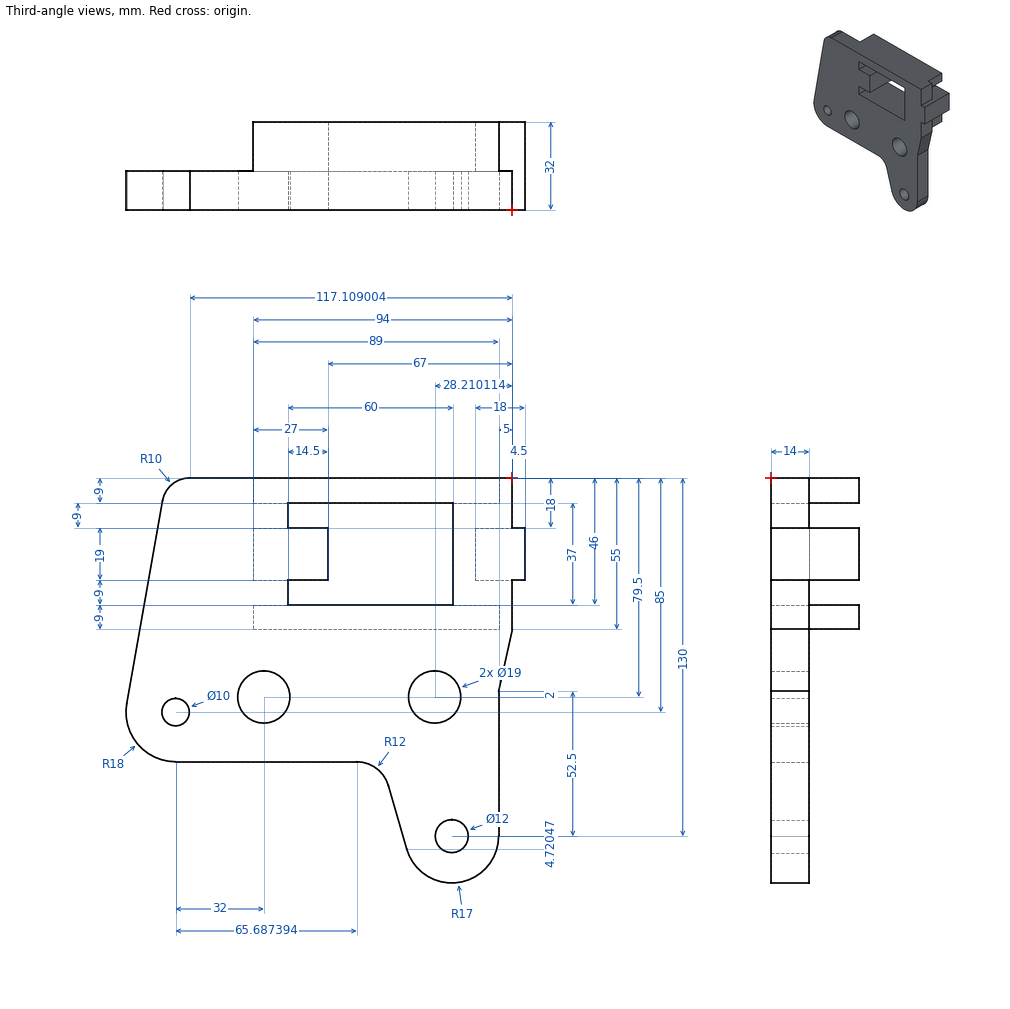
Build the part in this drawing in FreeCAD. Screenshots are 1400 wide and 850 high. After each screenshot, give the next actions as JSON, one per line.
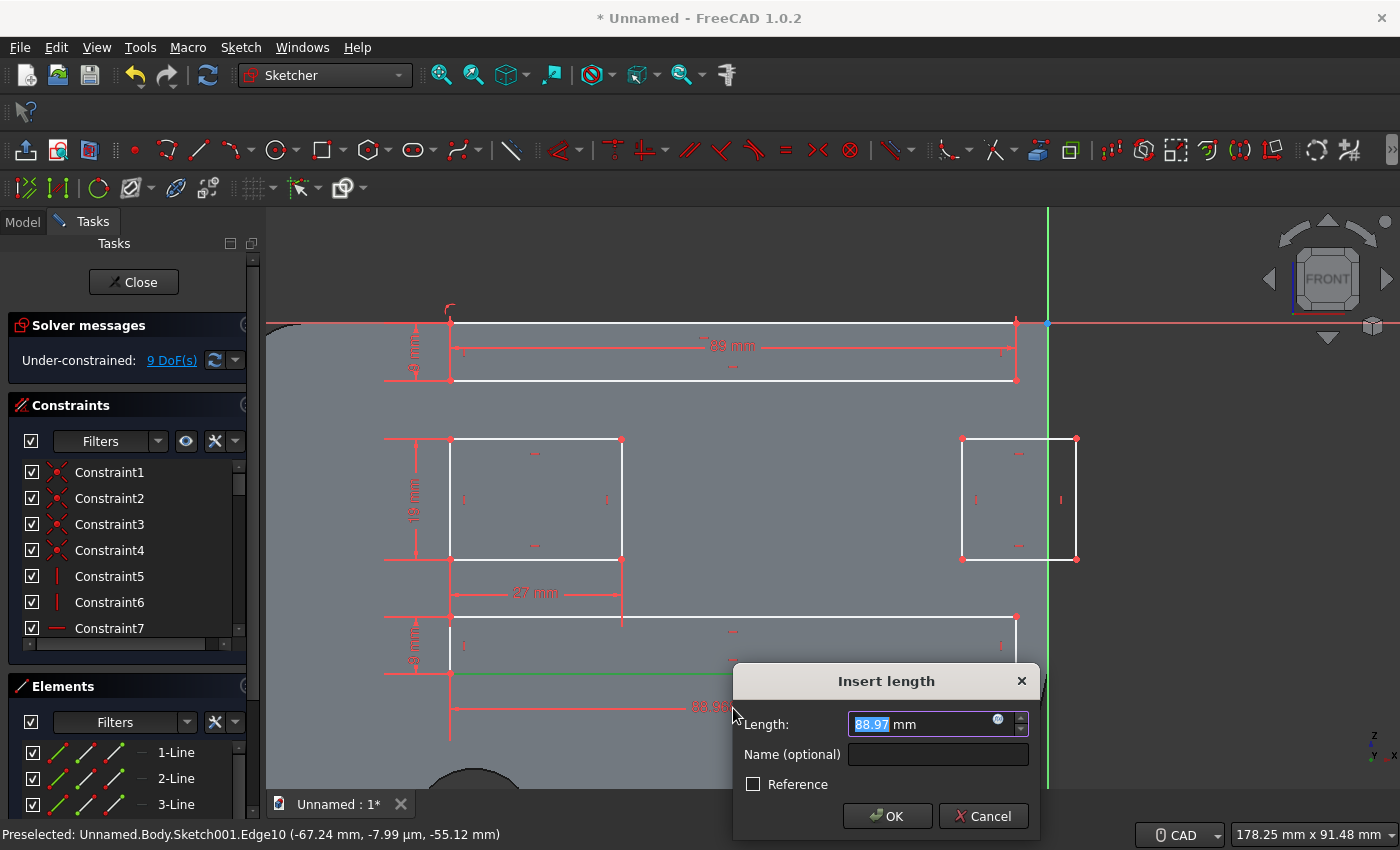
{"action": "type", "text": "89"}
{"action": "key", "text": "Return"}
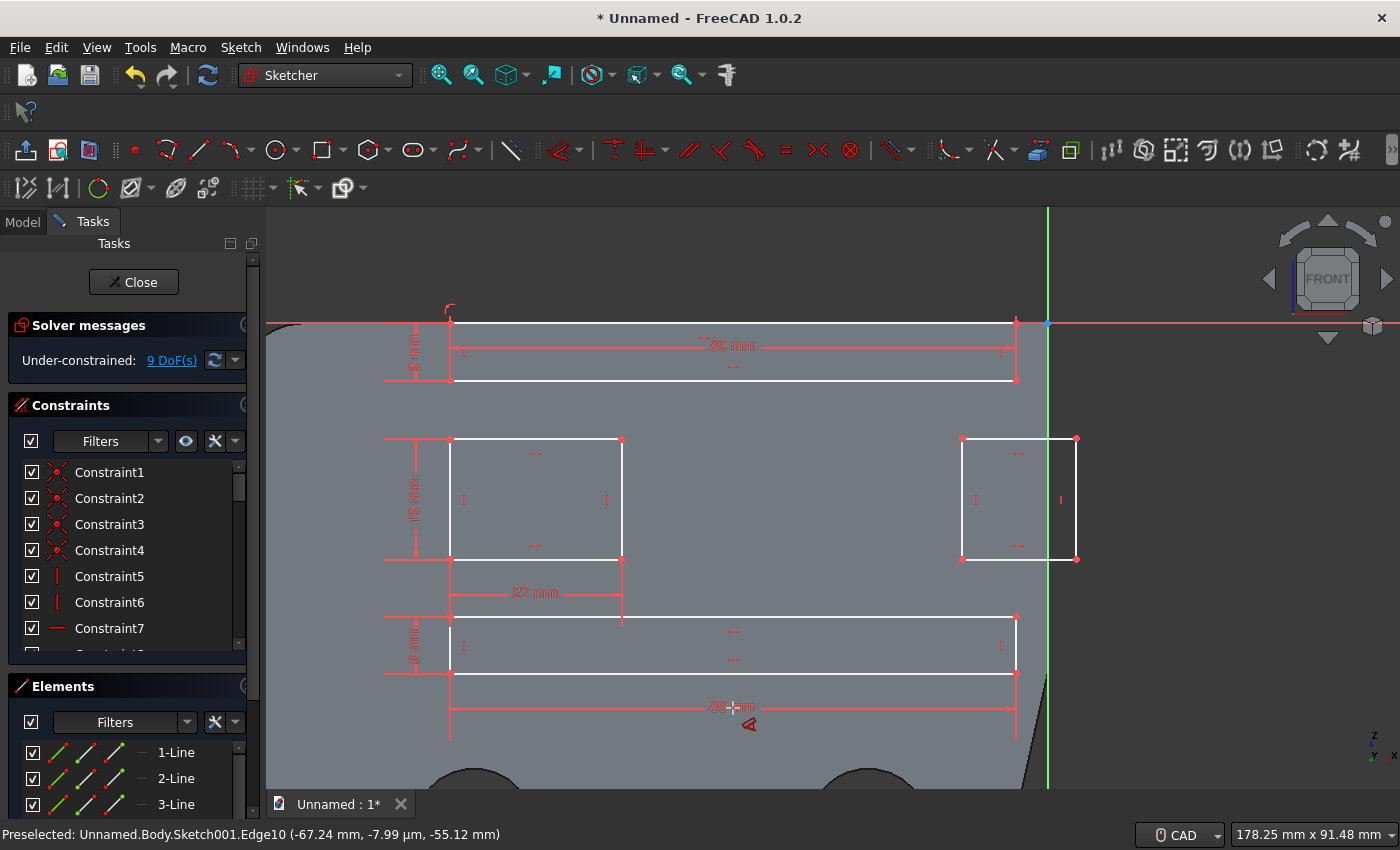
{"action": "left_click", "coordinate": [962, 475]}
{"action": "left_click", "coordinate": [996, 500]}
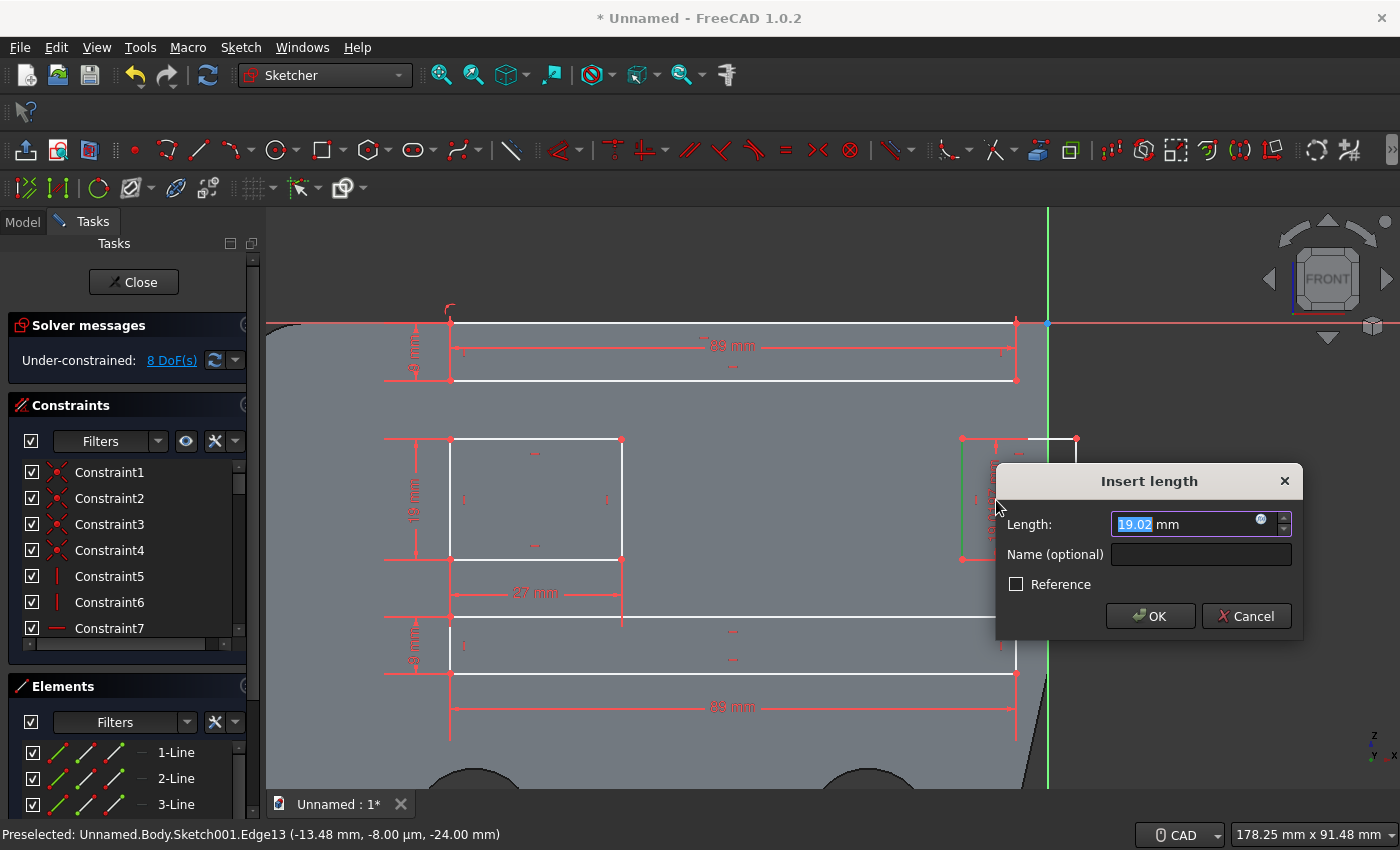
{"action": "type", "text": "19"}
{"action": "key", "text": "Return"}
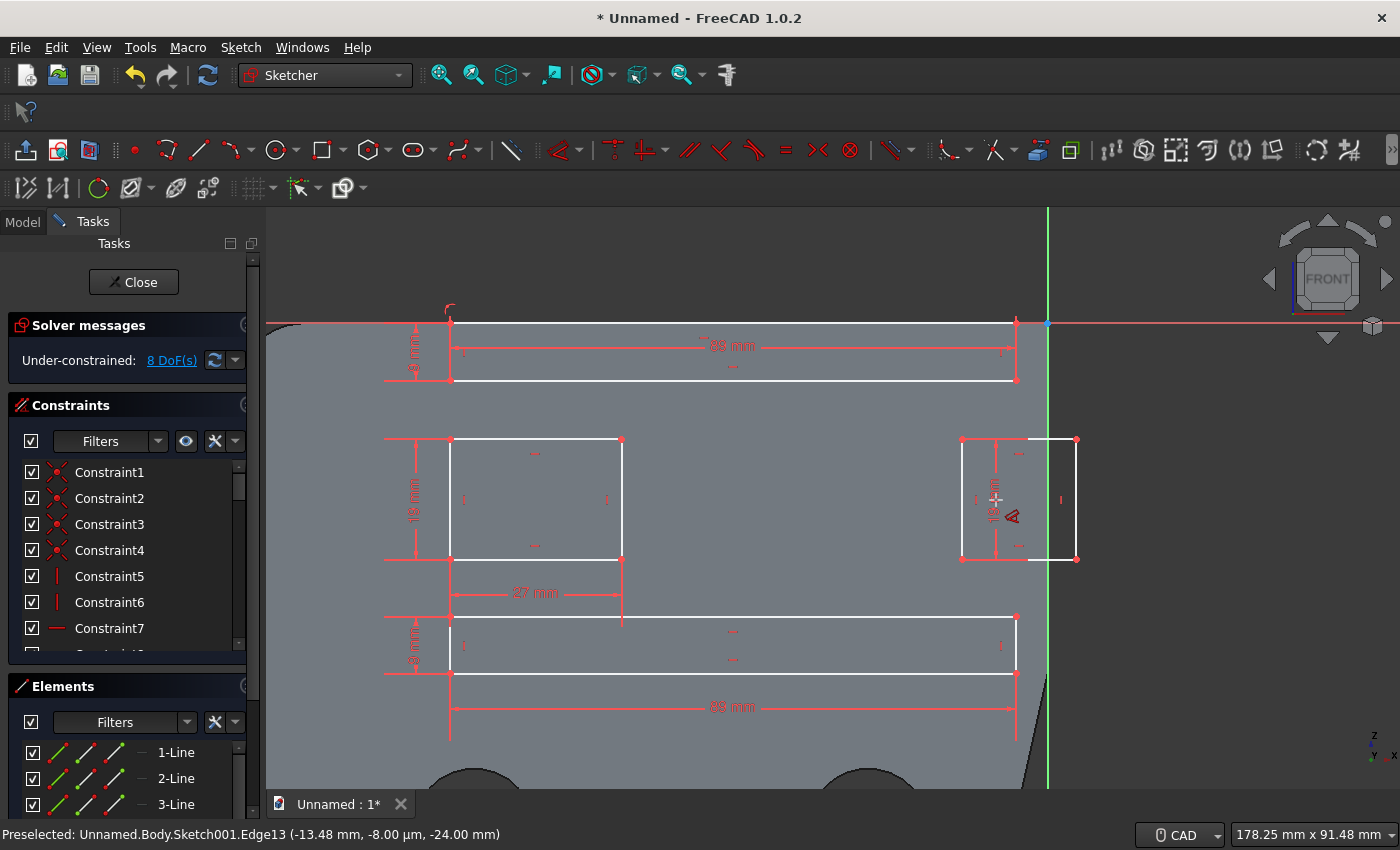
{"action": "left_click", "coordinate": [996, 560]}
{"action": "left_click", "coordinate": [1019, 594]}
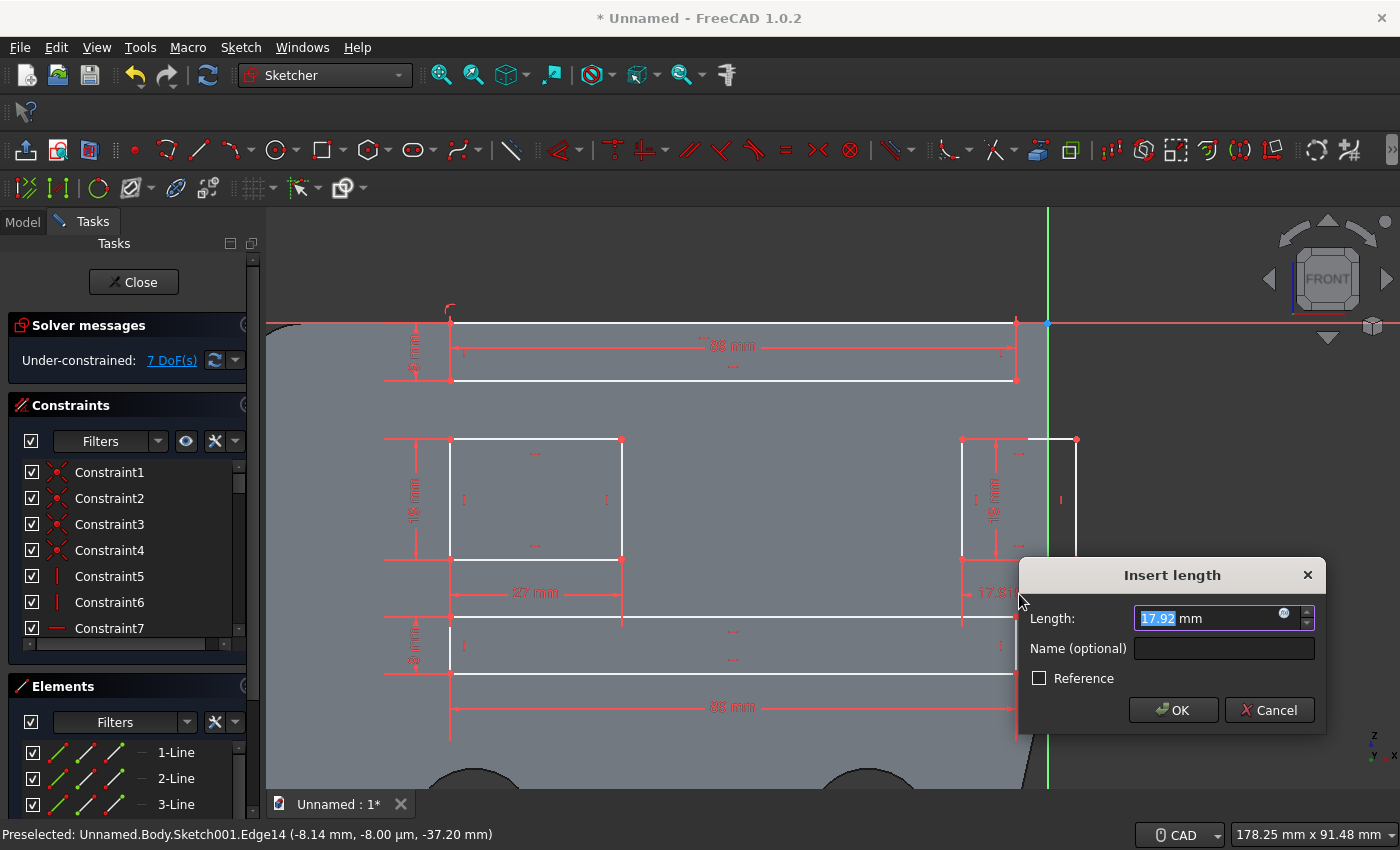
{"action": "type", "text": "18"}
{"action": "key", "text": "Return"}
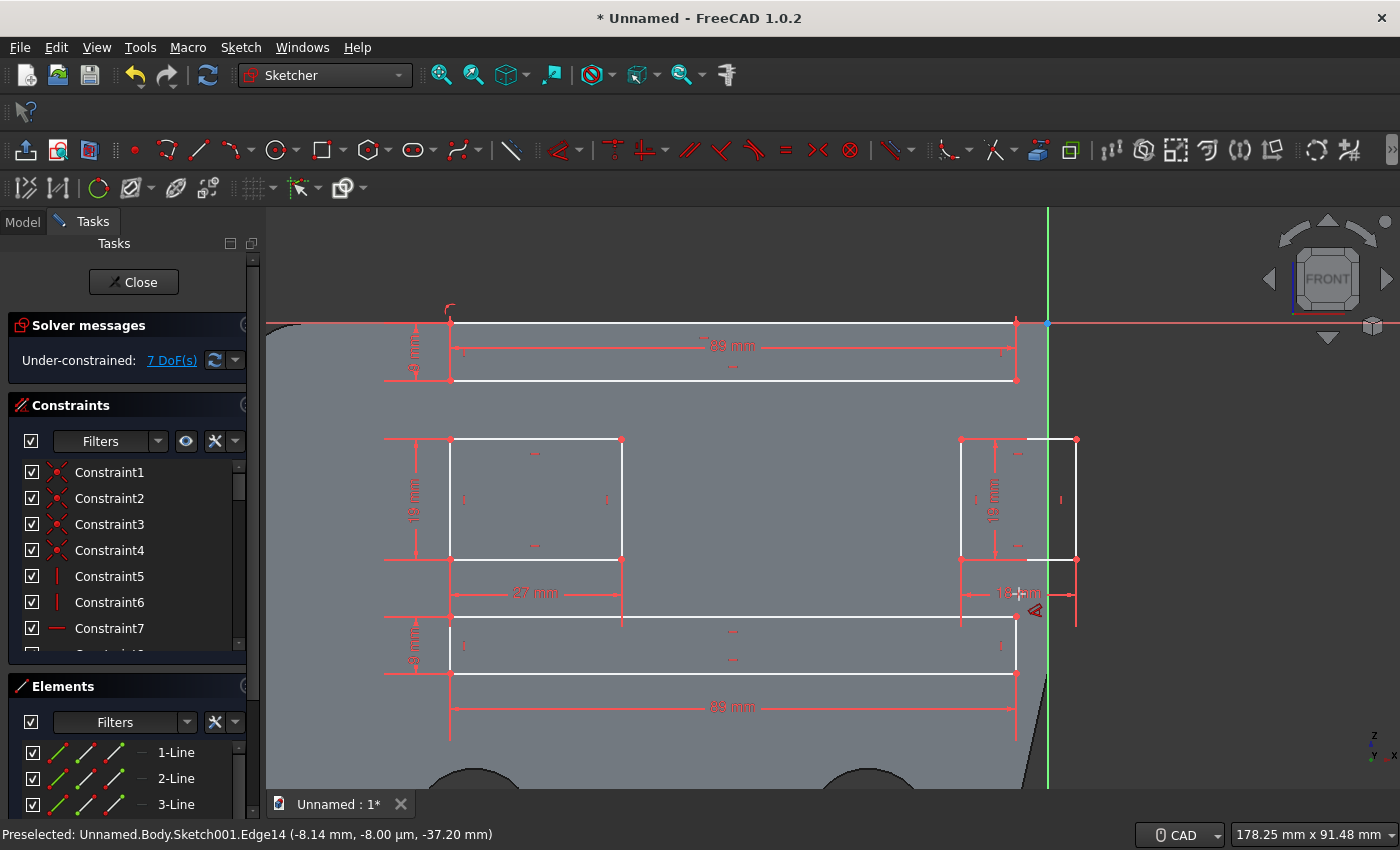
{"action": "scroll", "coordinate": [1016, 381], "scroll_direction": "up", "scroll_amount": 2}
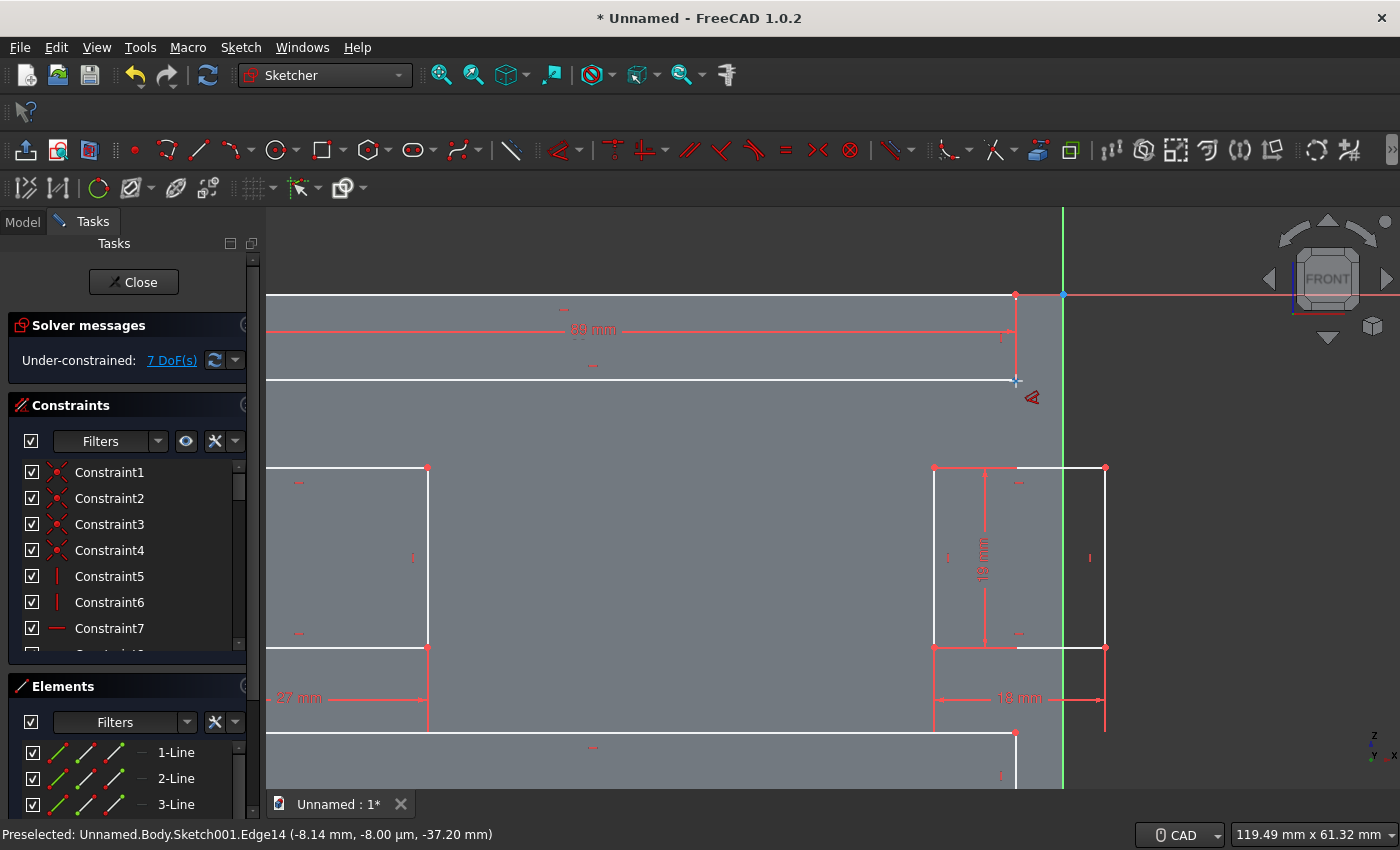
{"action": "left_click", "coordinate": [1016, 380]}
{"action": "left_click", "coordinate": [1040, 261]}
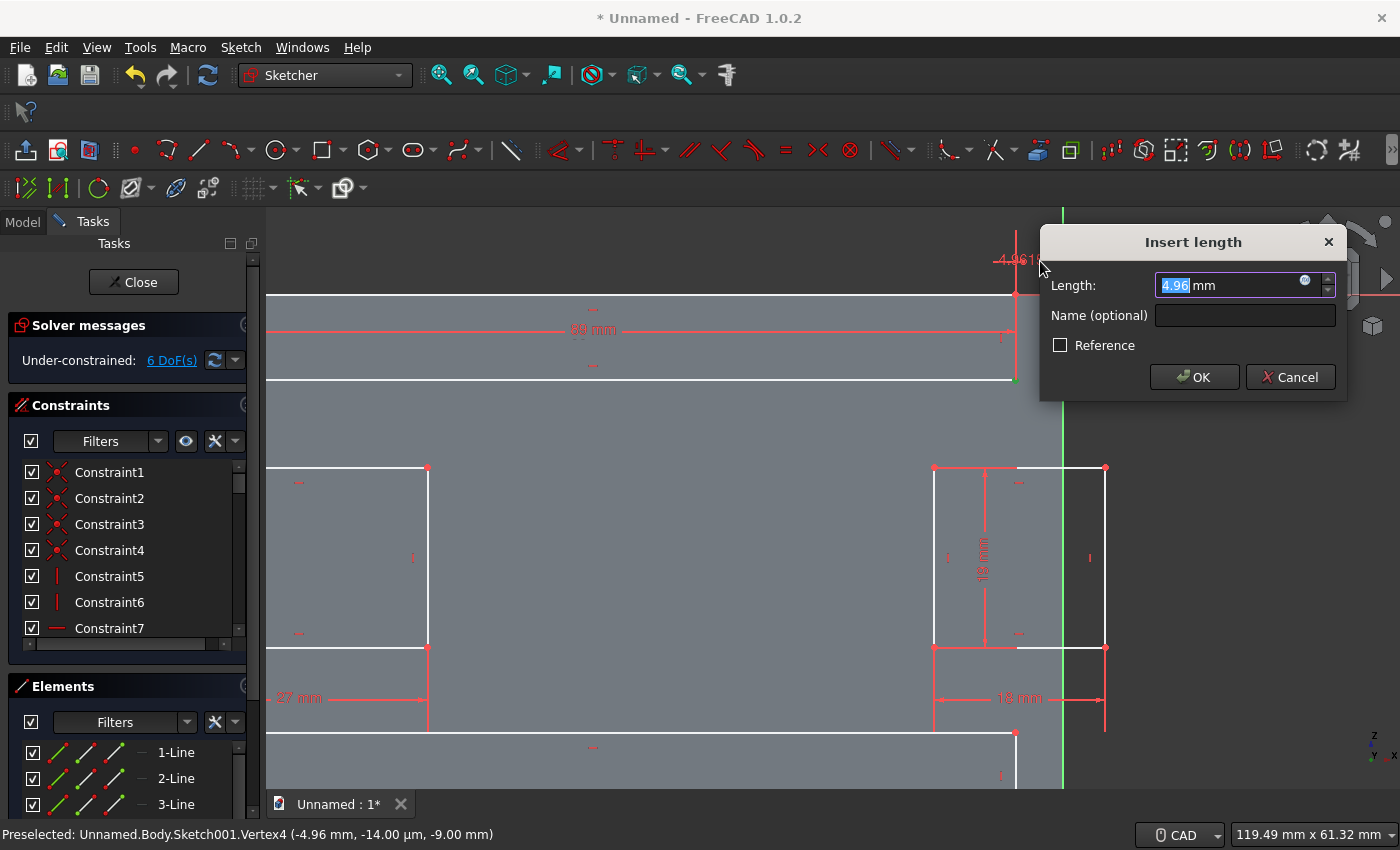
{"action": "type", "text": "5"}
{"action": "key", "text": "Return"}